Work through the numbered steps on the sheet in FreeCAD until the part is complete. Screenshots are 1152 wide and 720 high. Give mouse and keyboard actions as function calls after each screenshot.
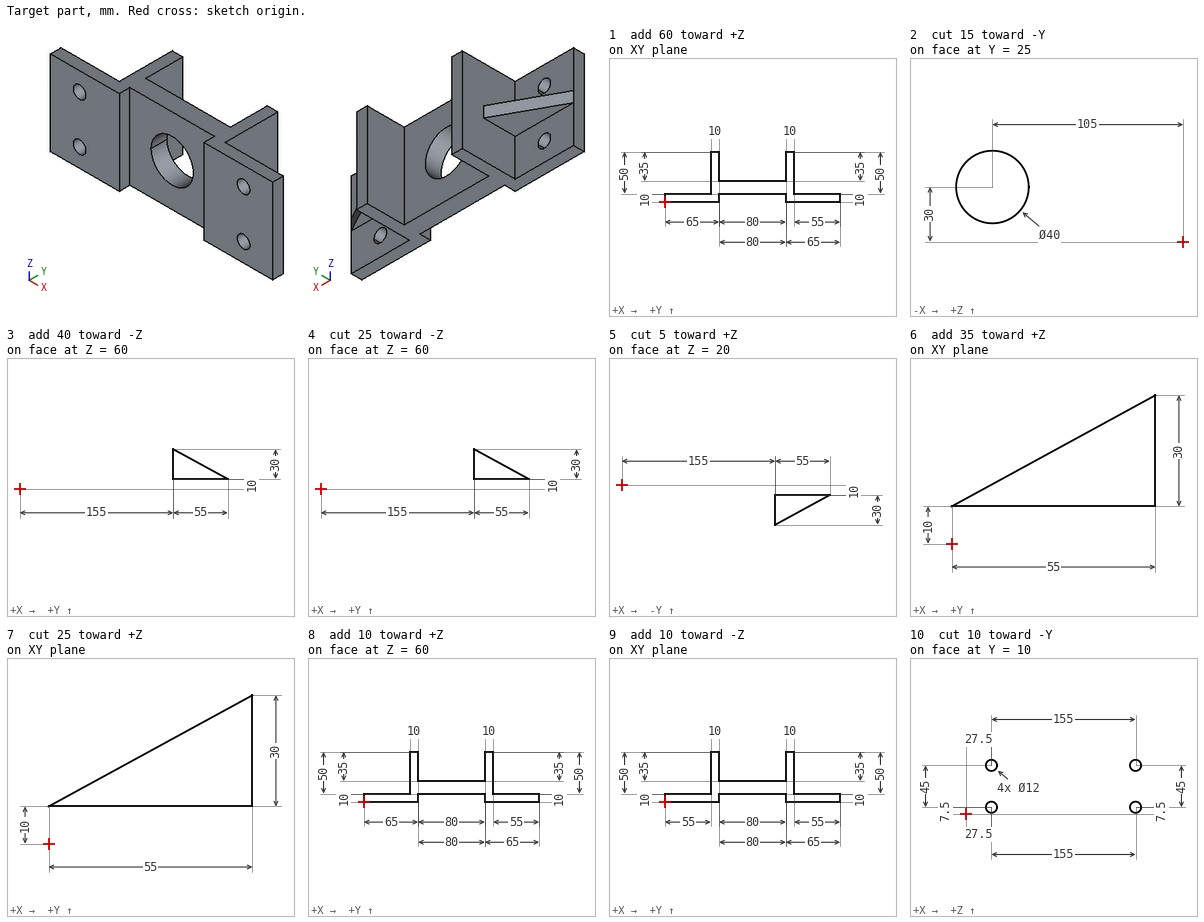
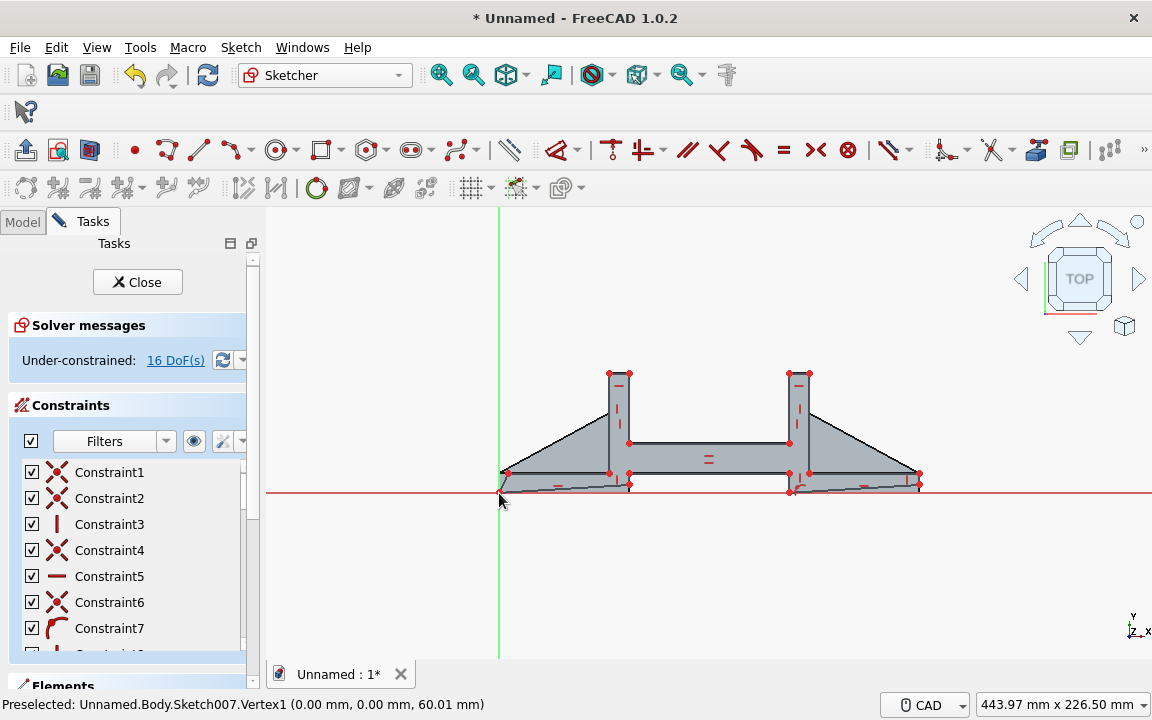
click(538, 491)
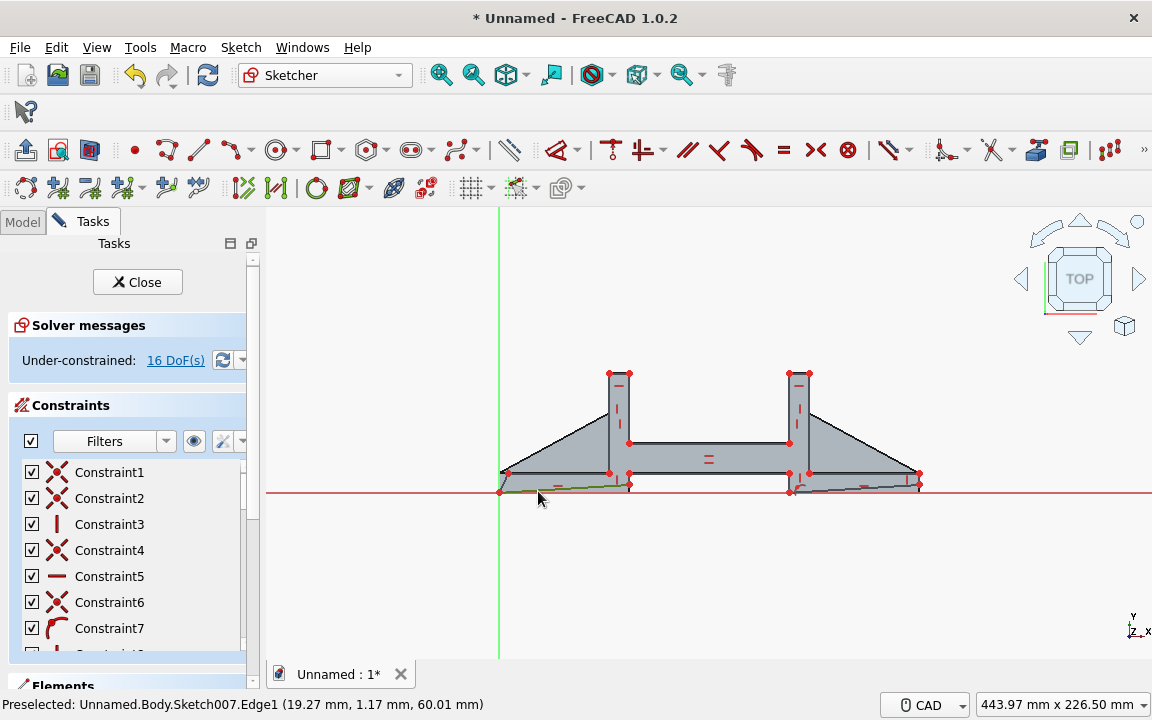
key(h)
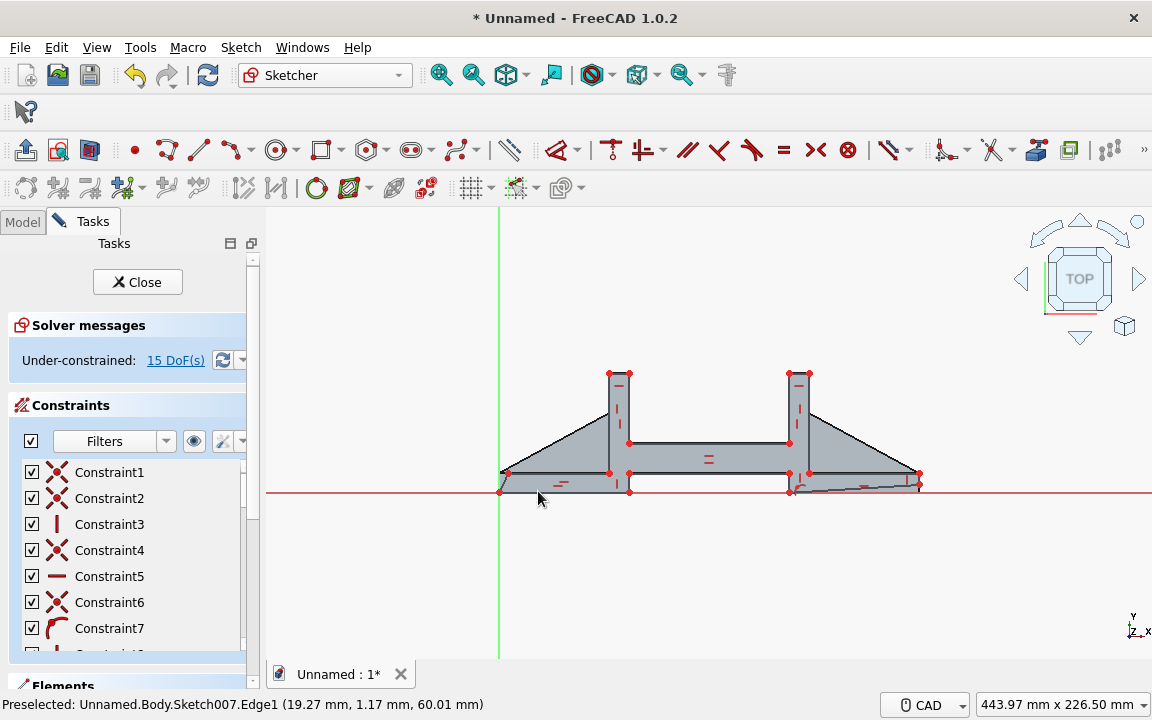
click(828, 491)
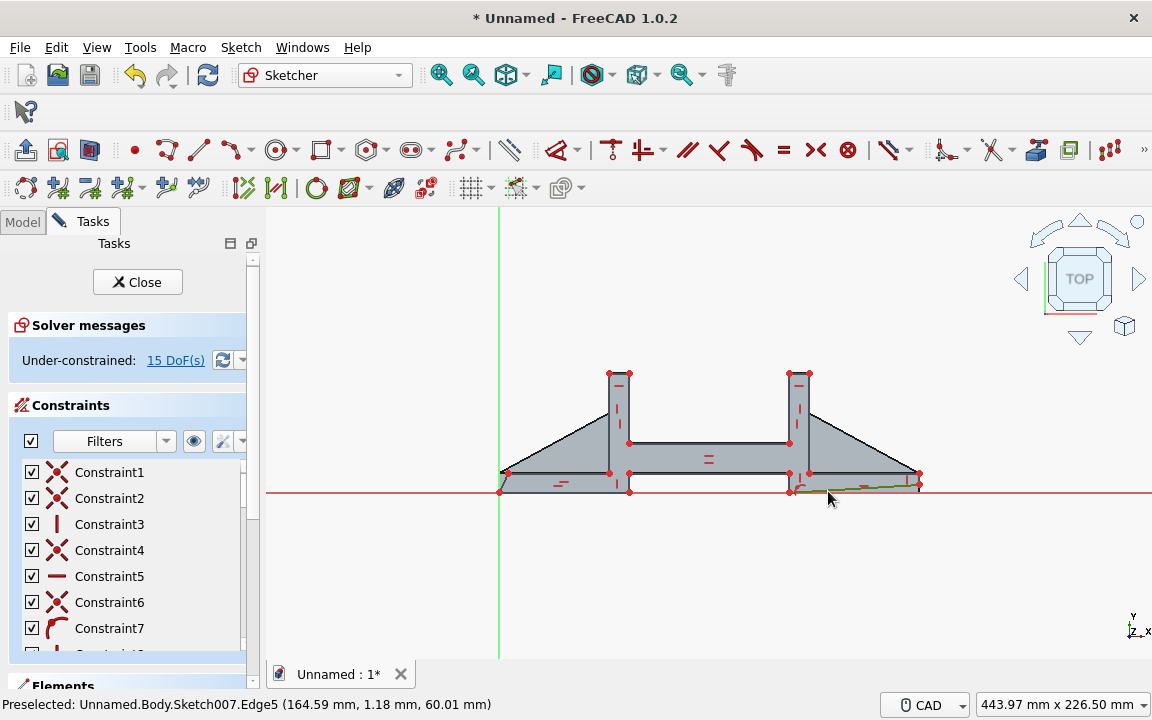
key(h)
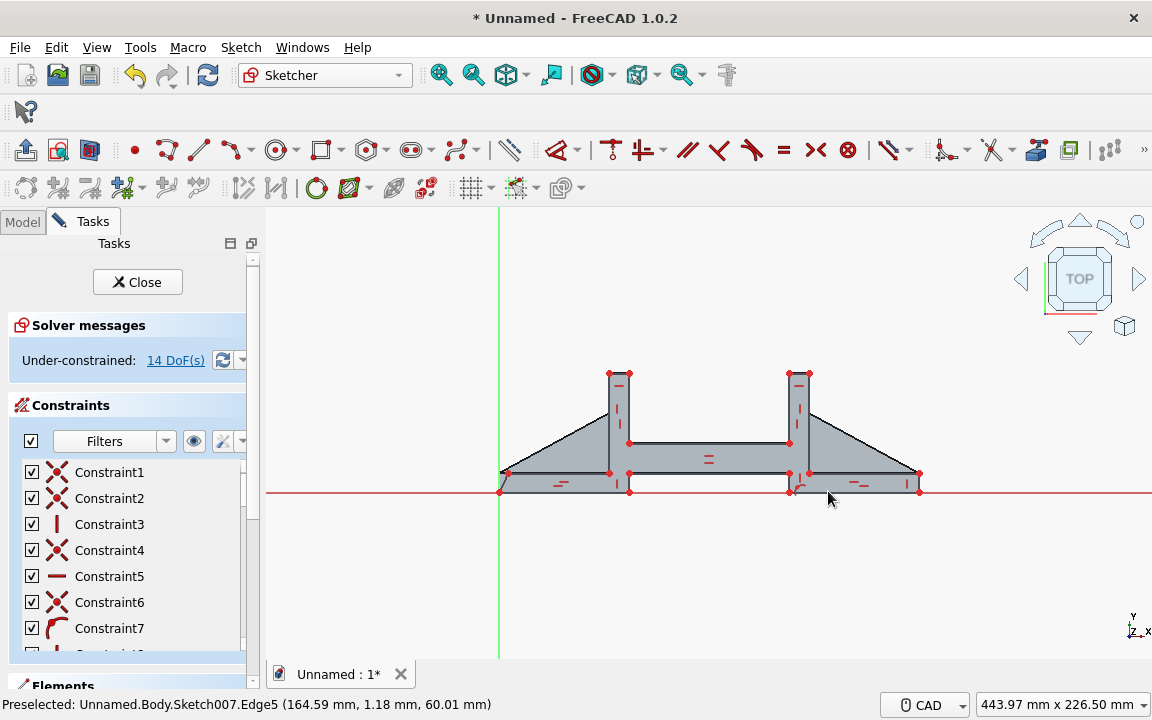
scroll(503, 485, up, 4)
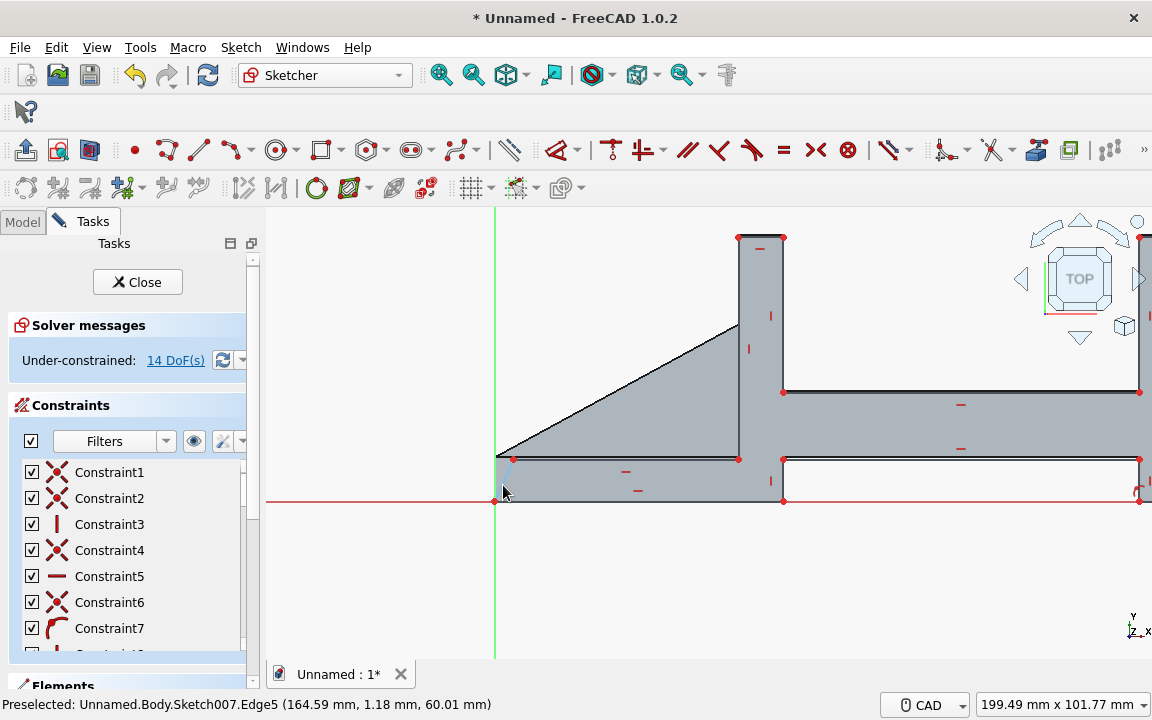
click(502, 485)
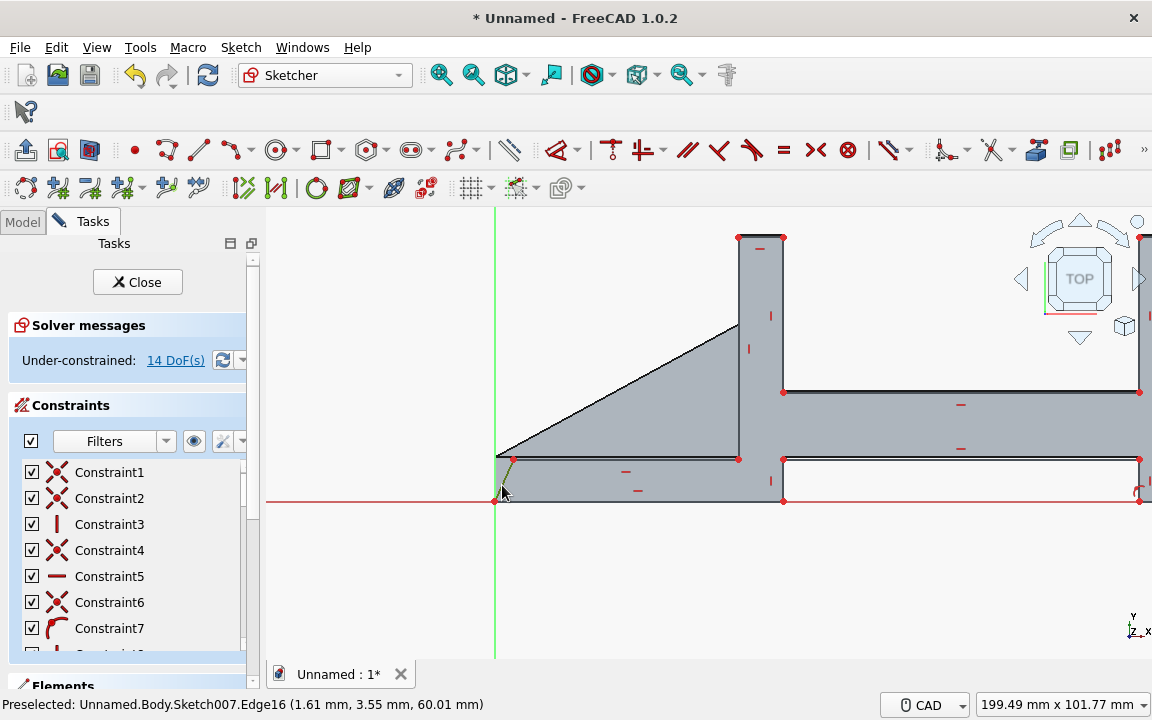
key(v)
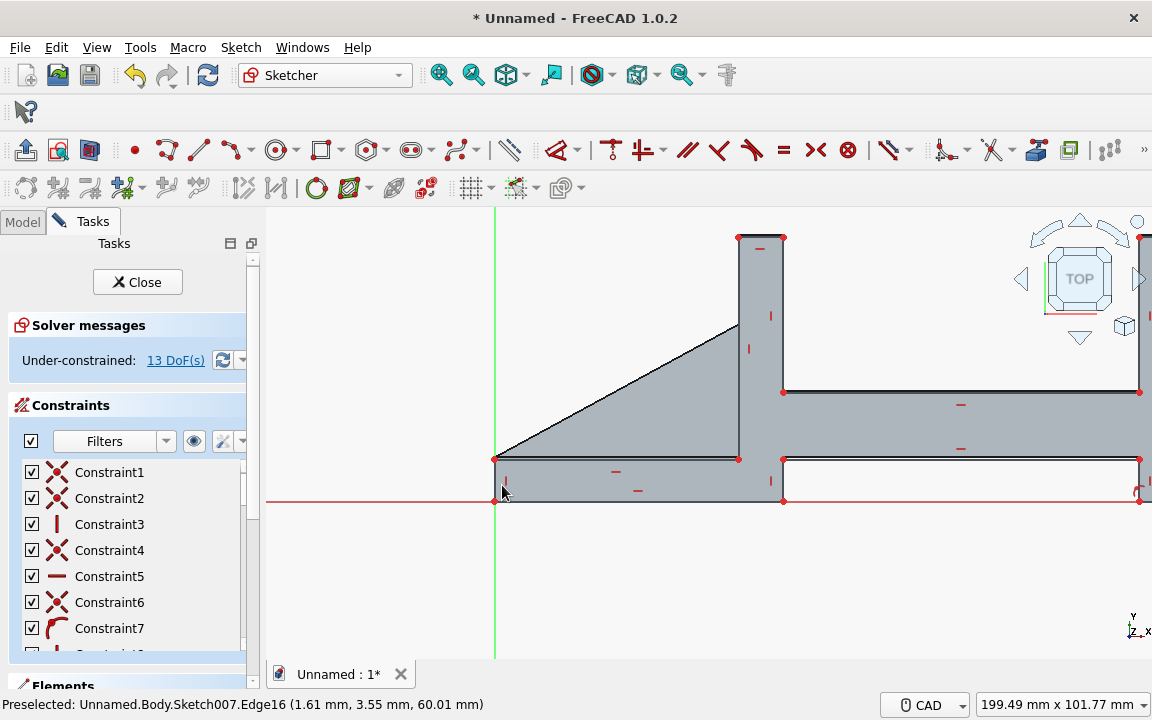
key(d)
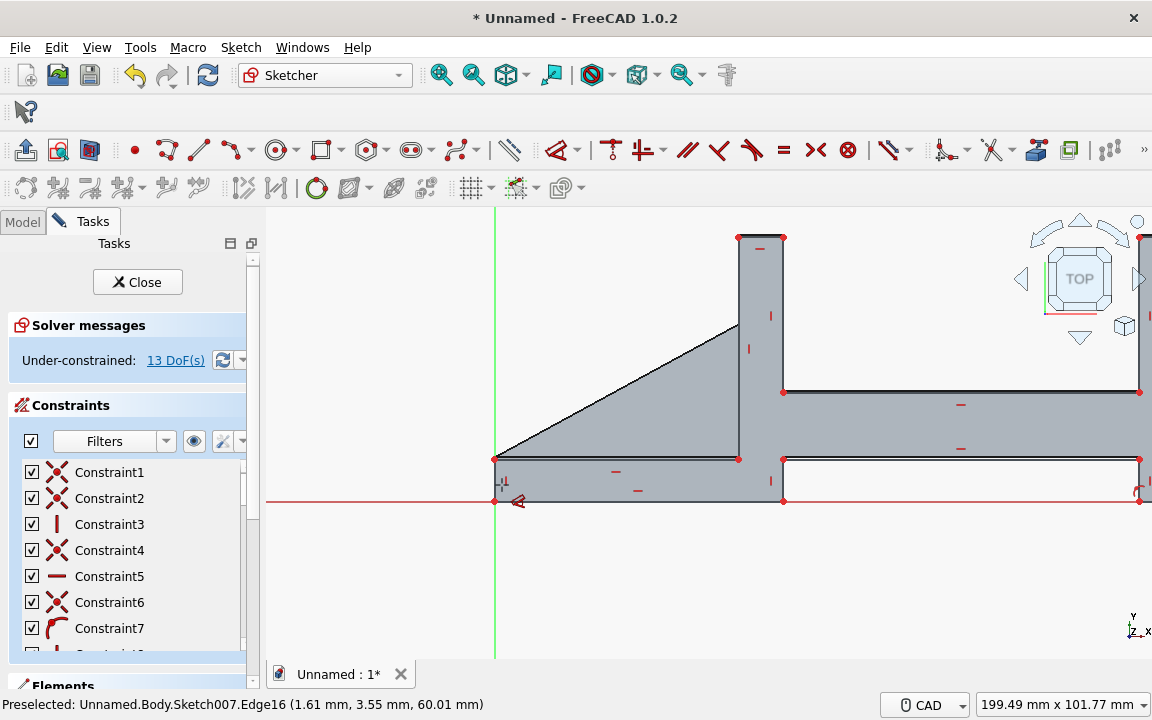
click(581, 502)
click(639, 536)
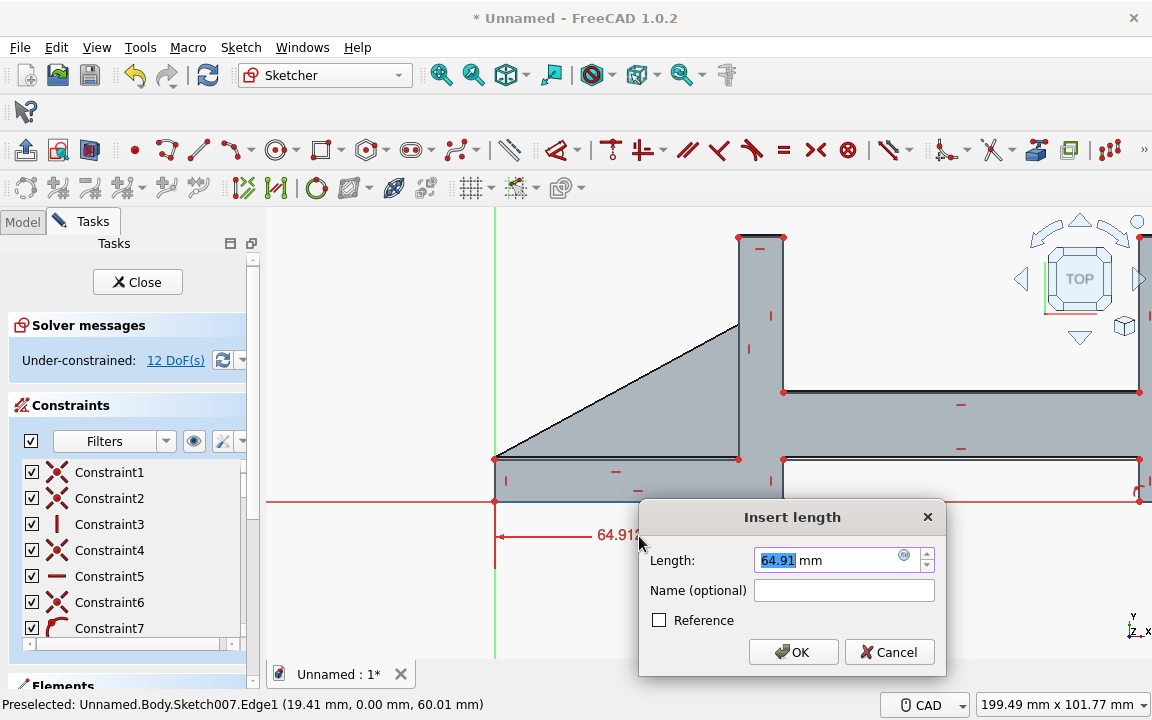
text(65)
key(Return)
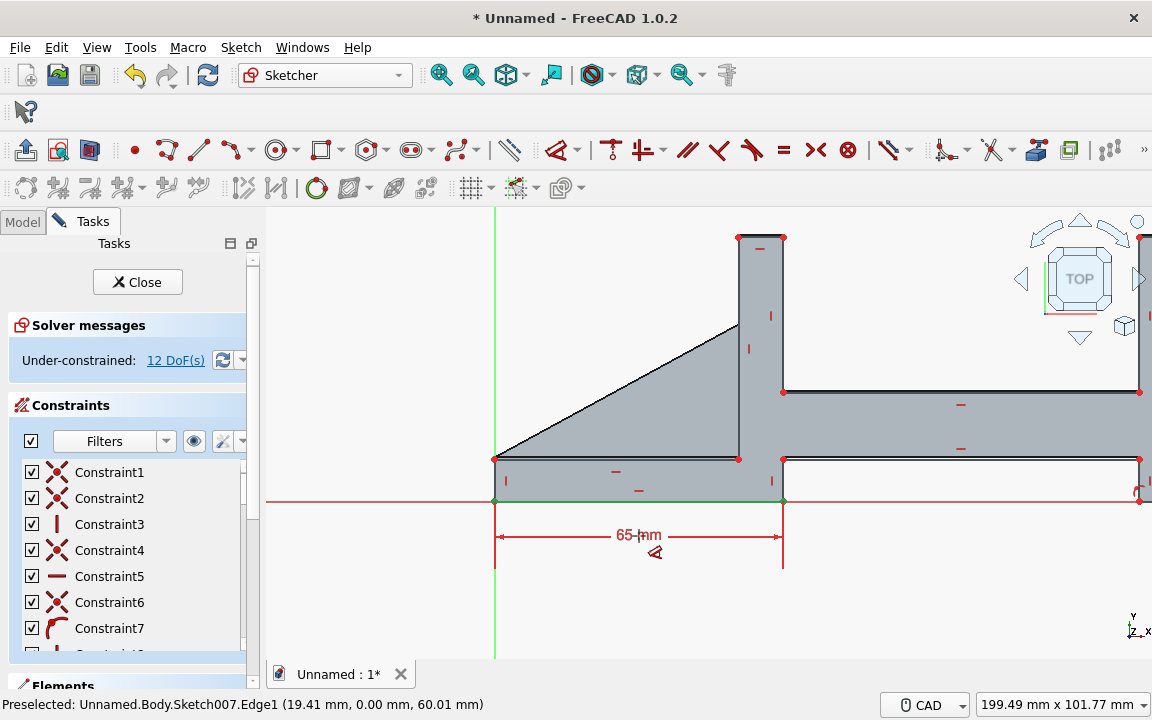
click(783, 489)
click(749, 481)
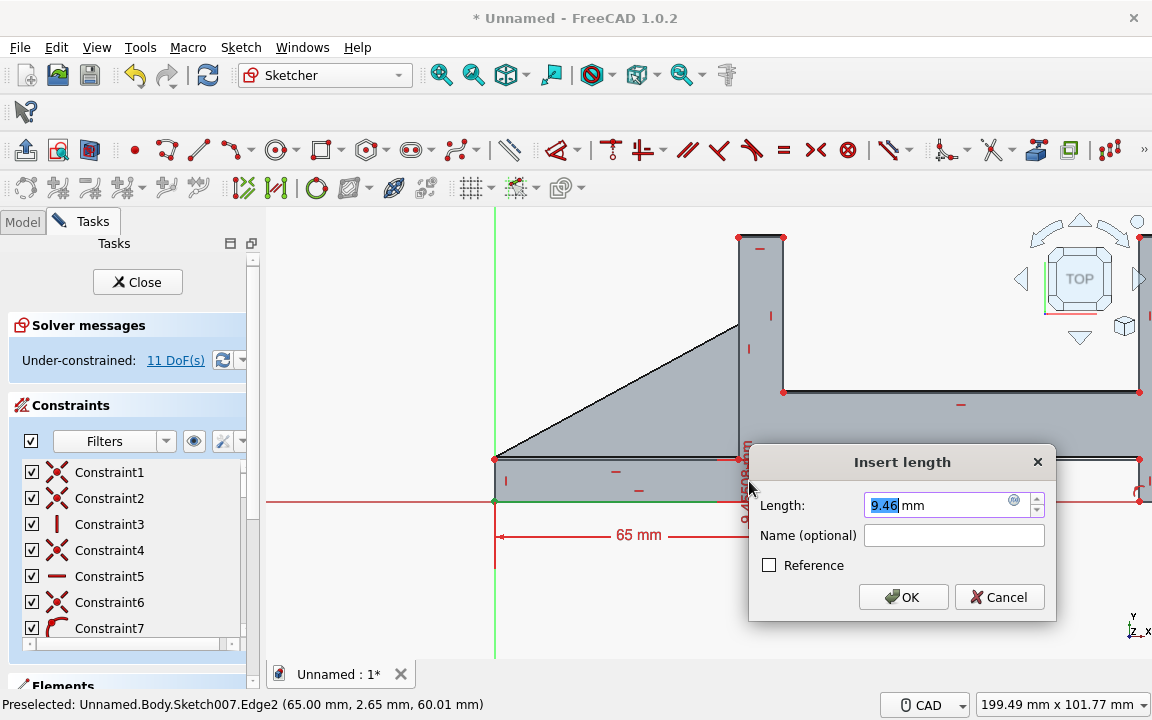
text(10)
key(Return)